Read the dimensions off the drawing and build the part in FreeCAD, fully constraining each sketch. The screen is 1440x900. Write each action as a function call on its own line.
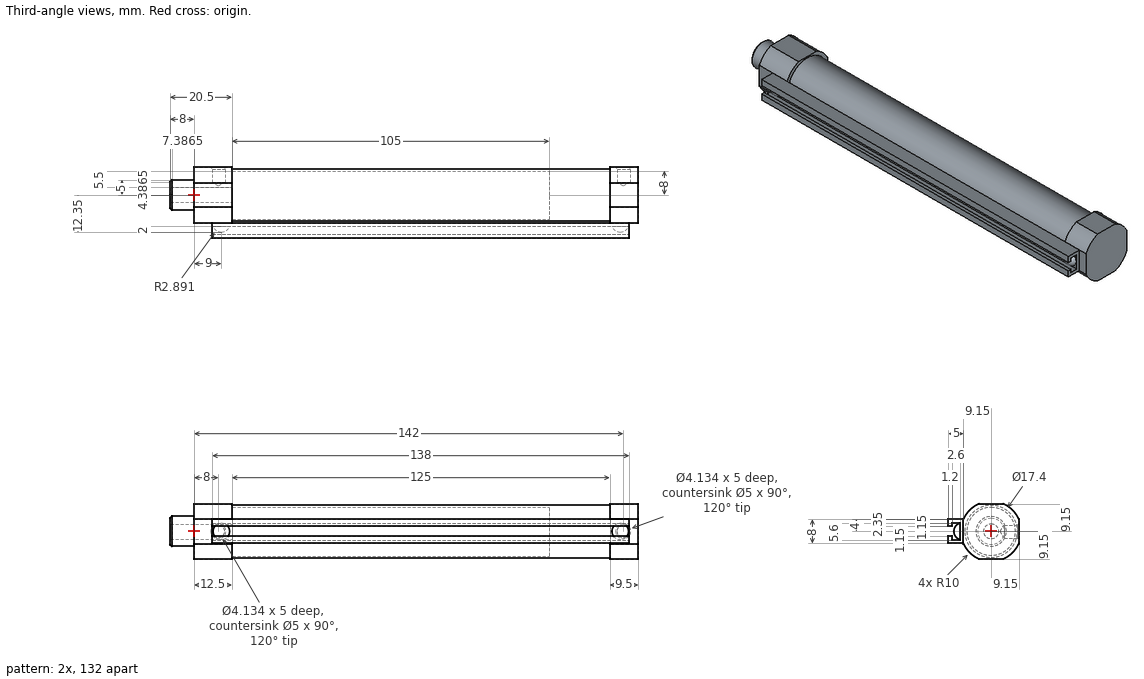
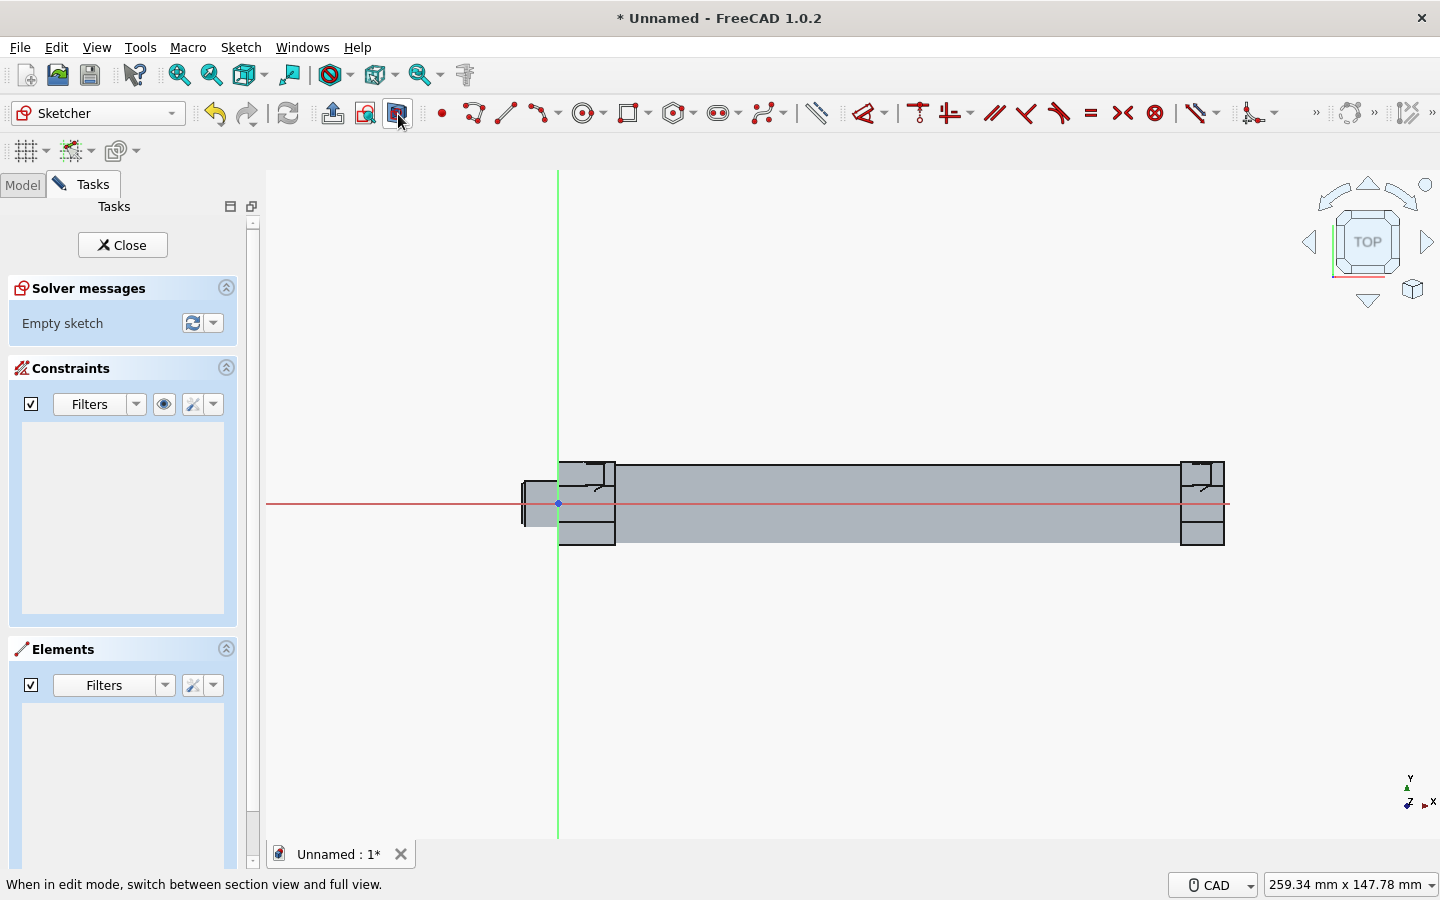
click(474, 114)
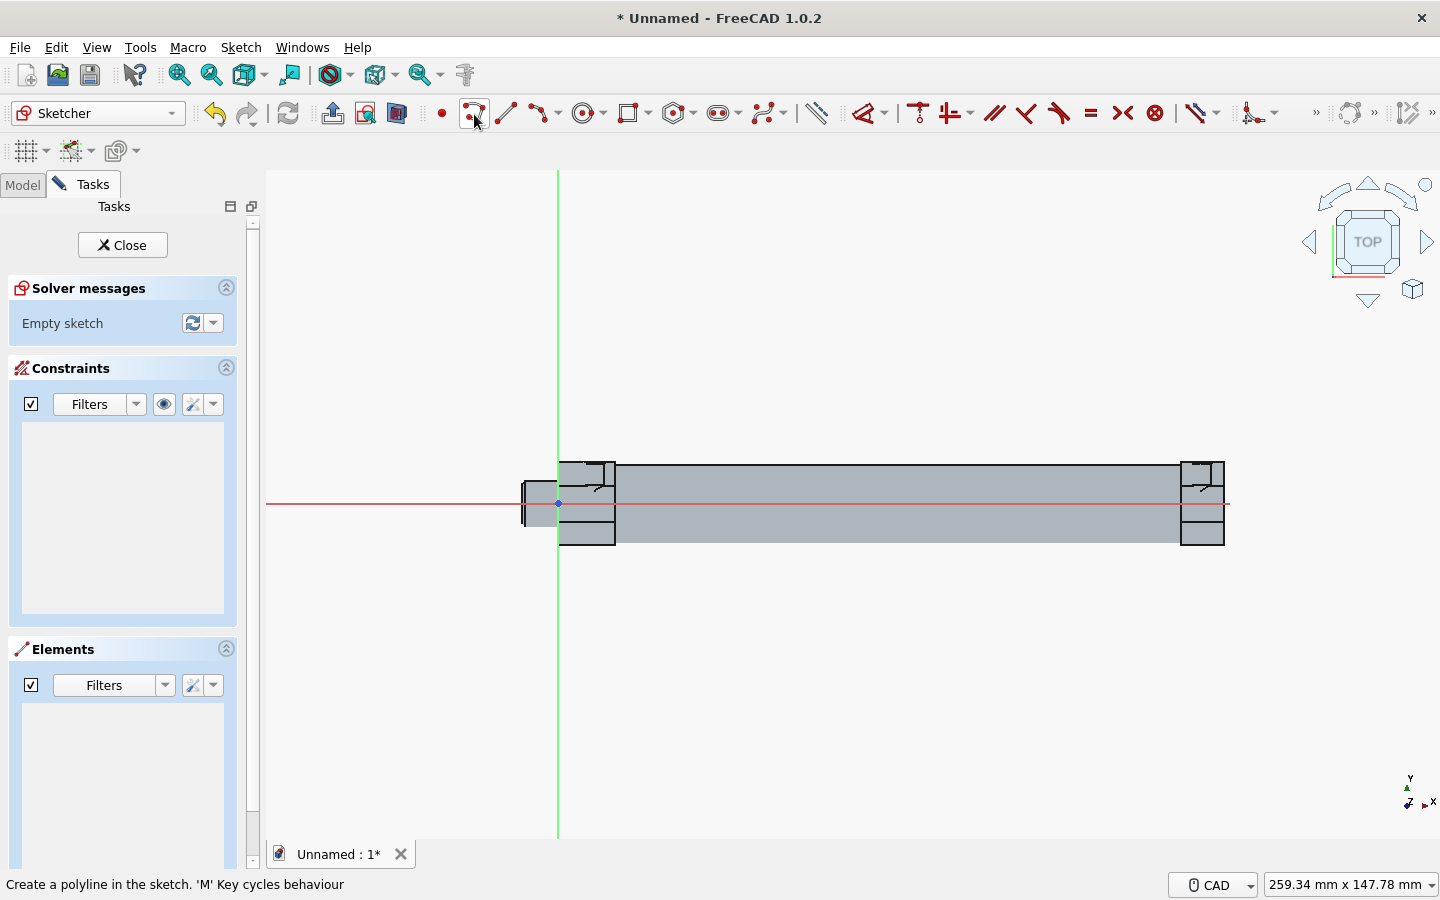
click(522, 504)
click(1090, 495)
click(1090, 468)
click(615, 468)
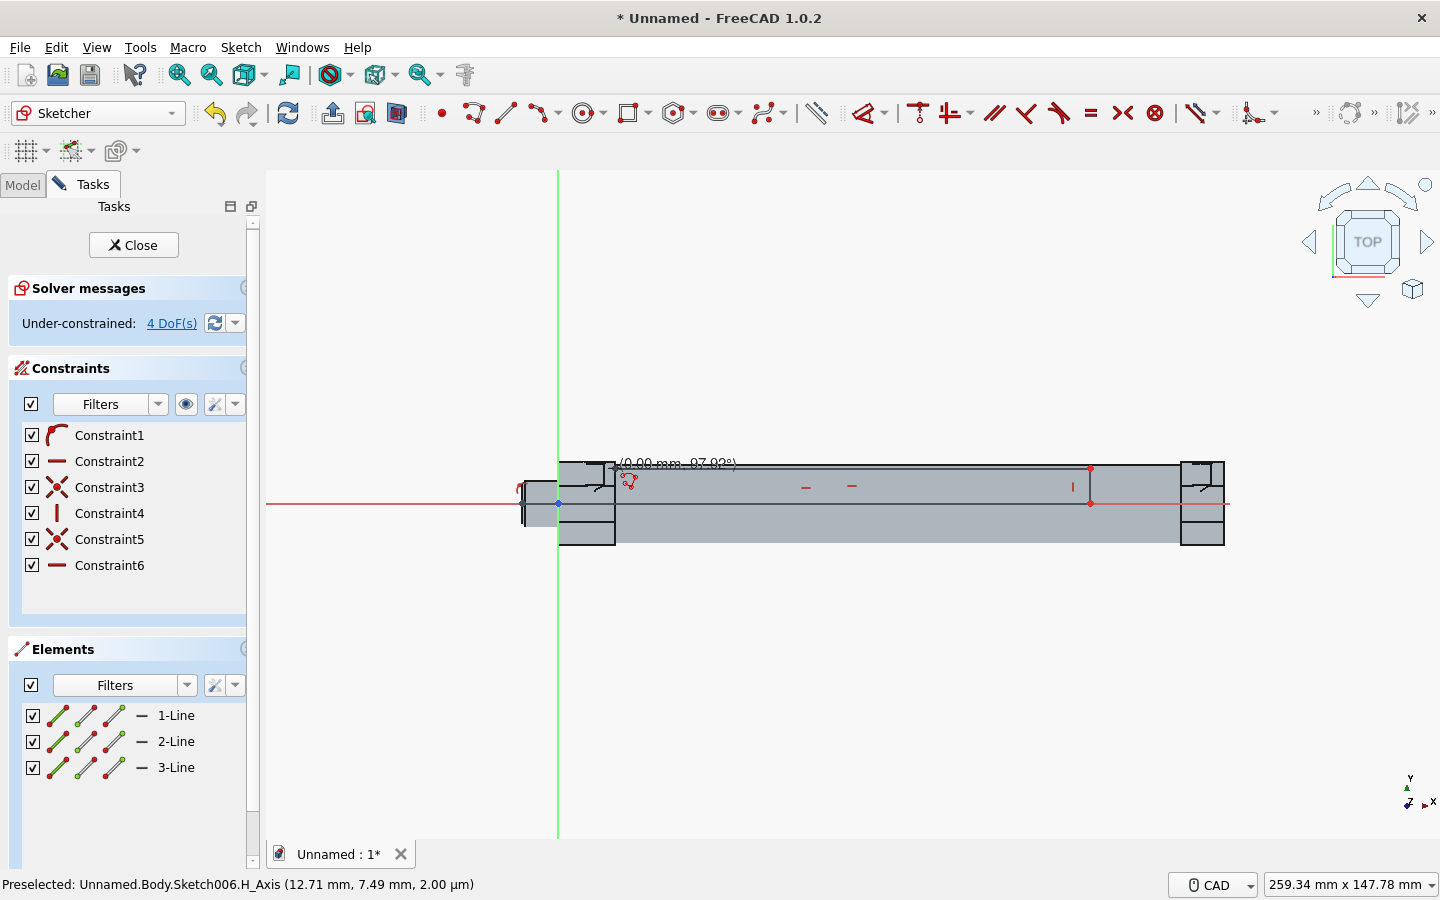
scroll(615, 493, up, 2)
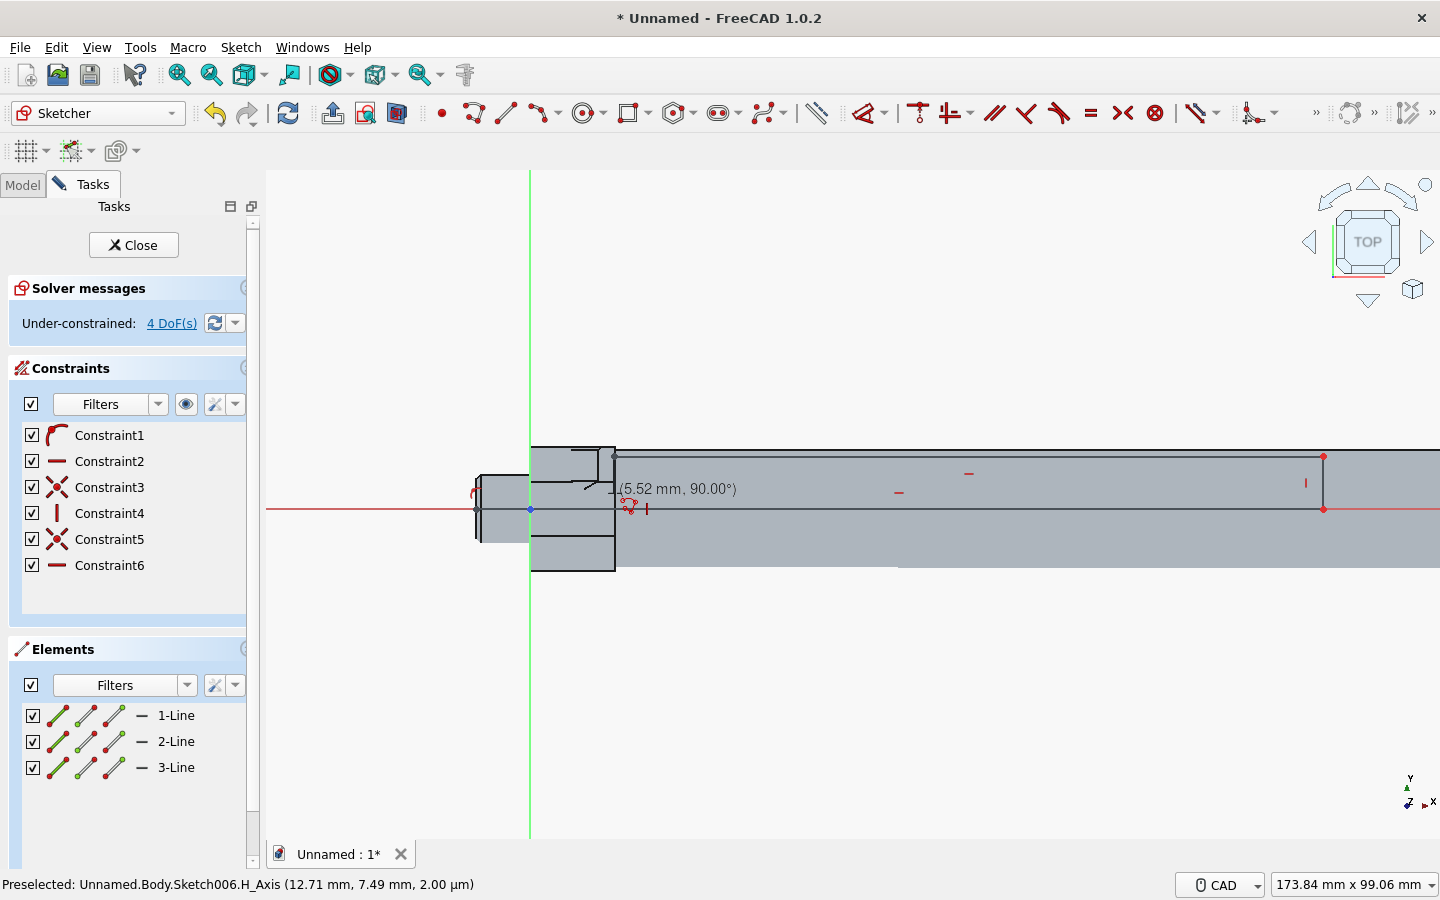
click(615, 492)
click(476, 492)
click(476, 509)
key(Escape)
key(Escape)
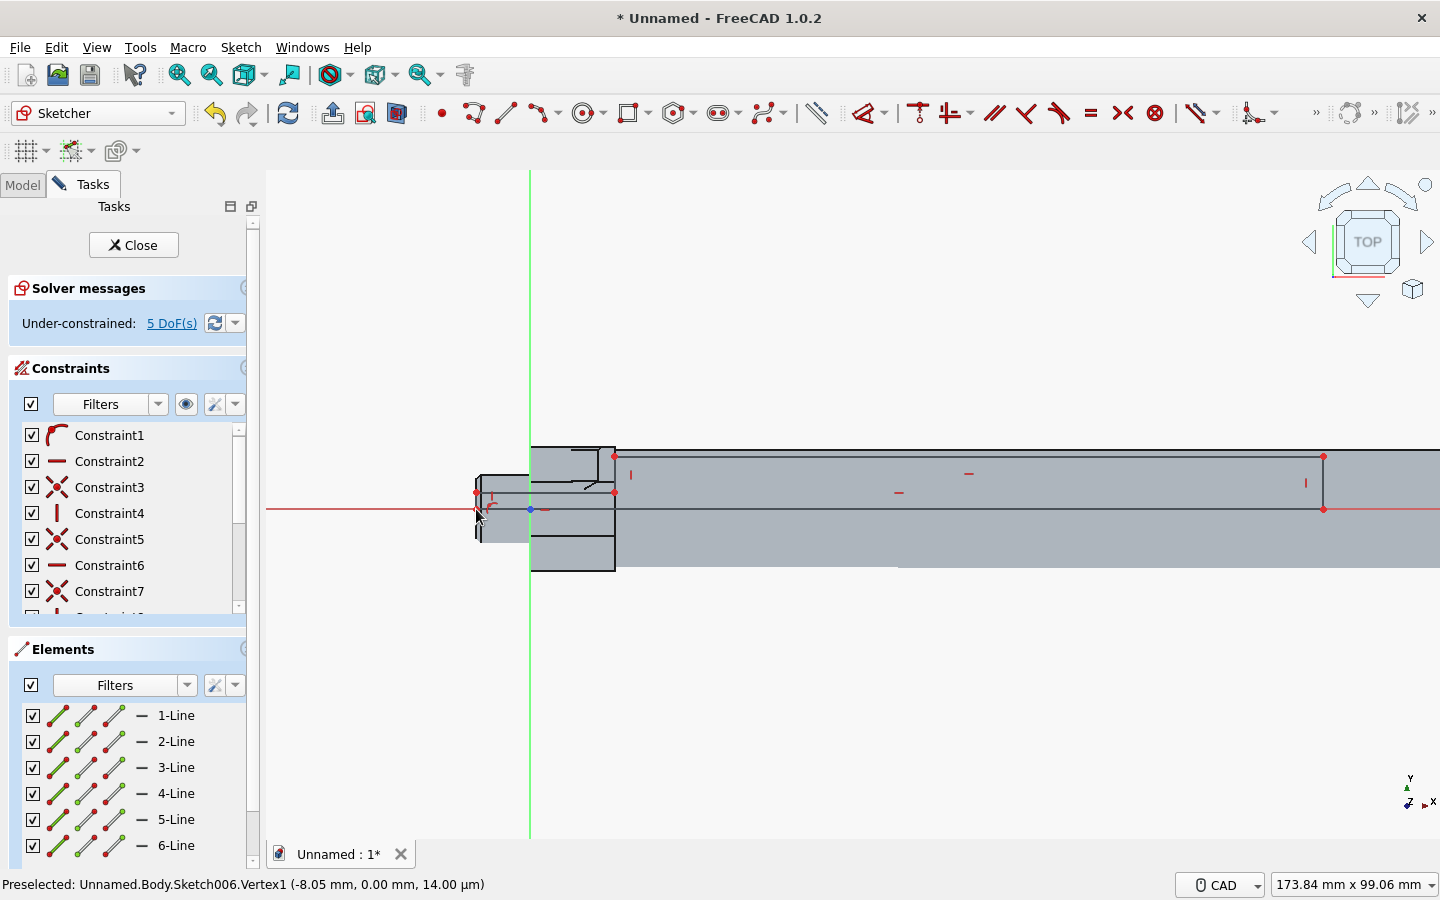
click(864, 114)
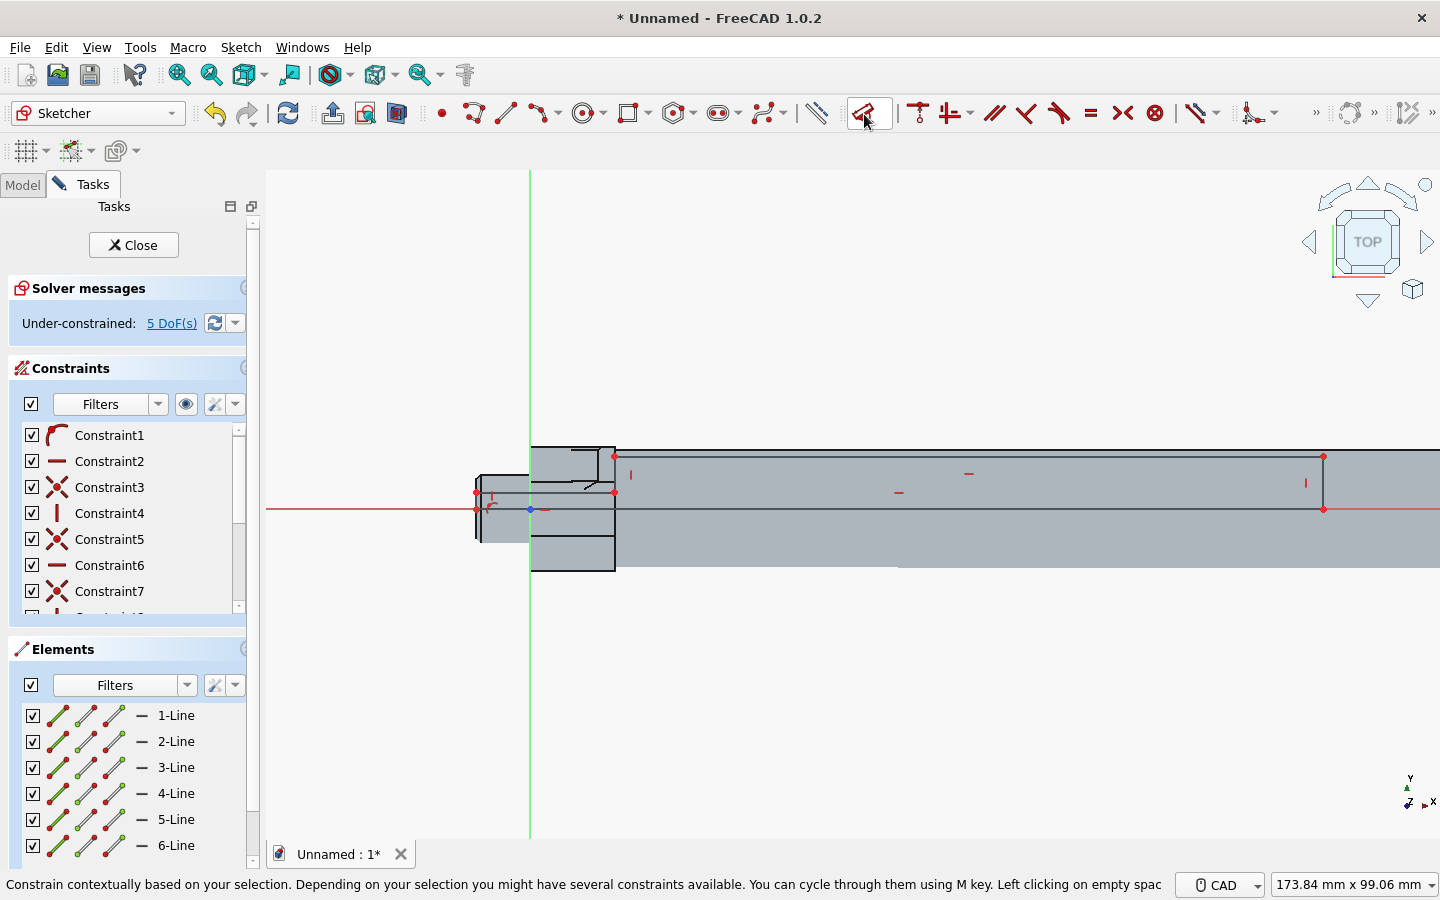
scroll(294, 606, down, 1)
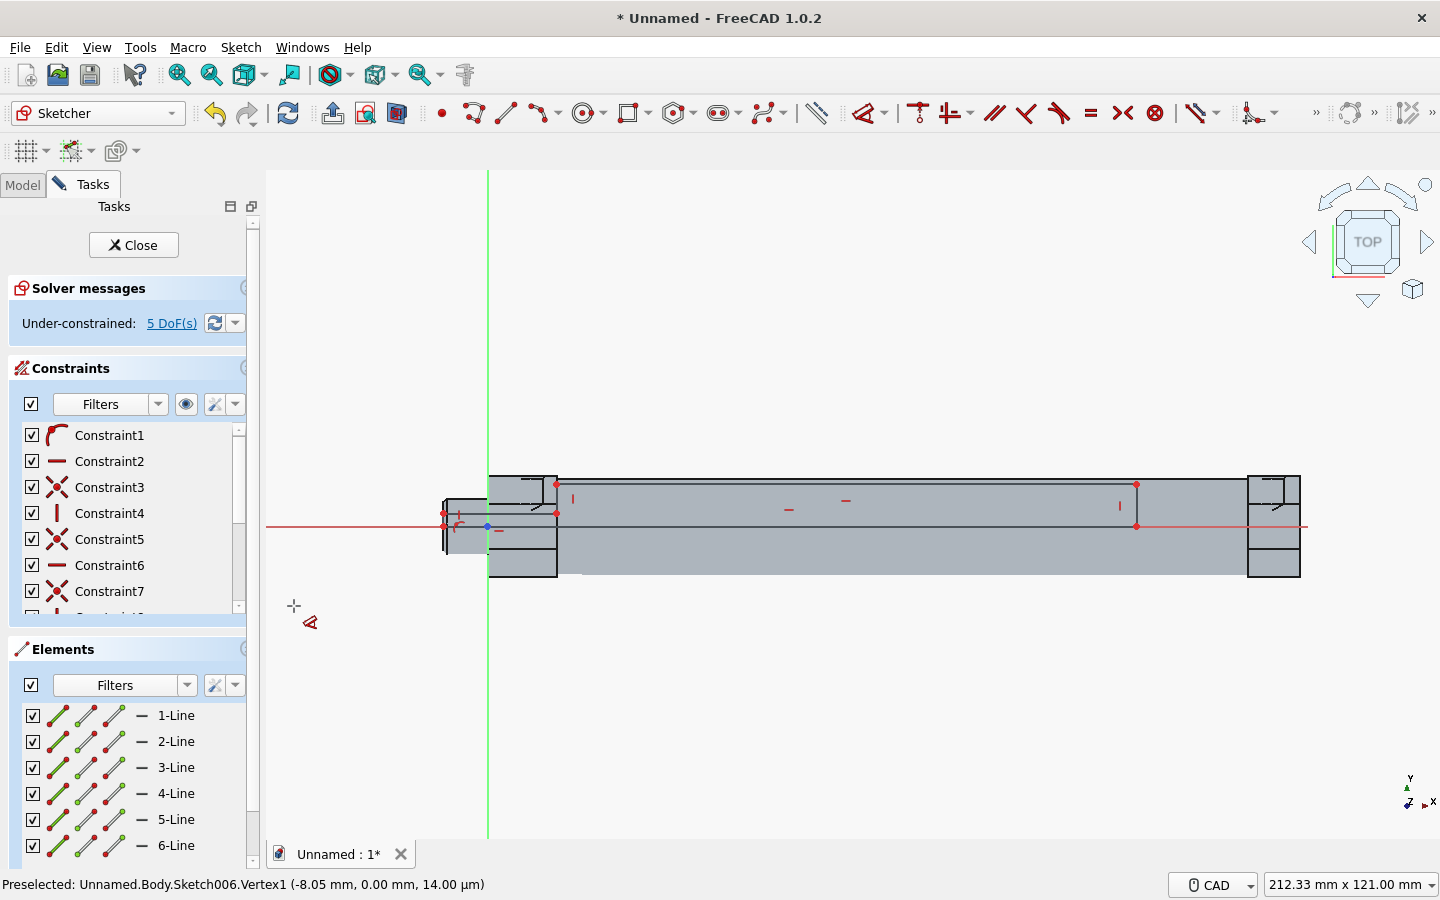
click(1137, 514)
click(1171, 505)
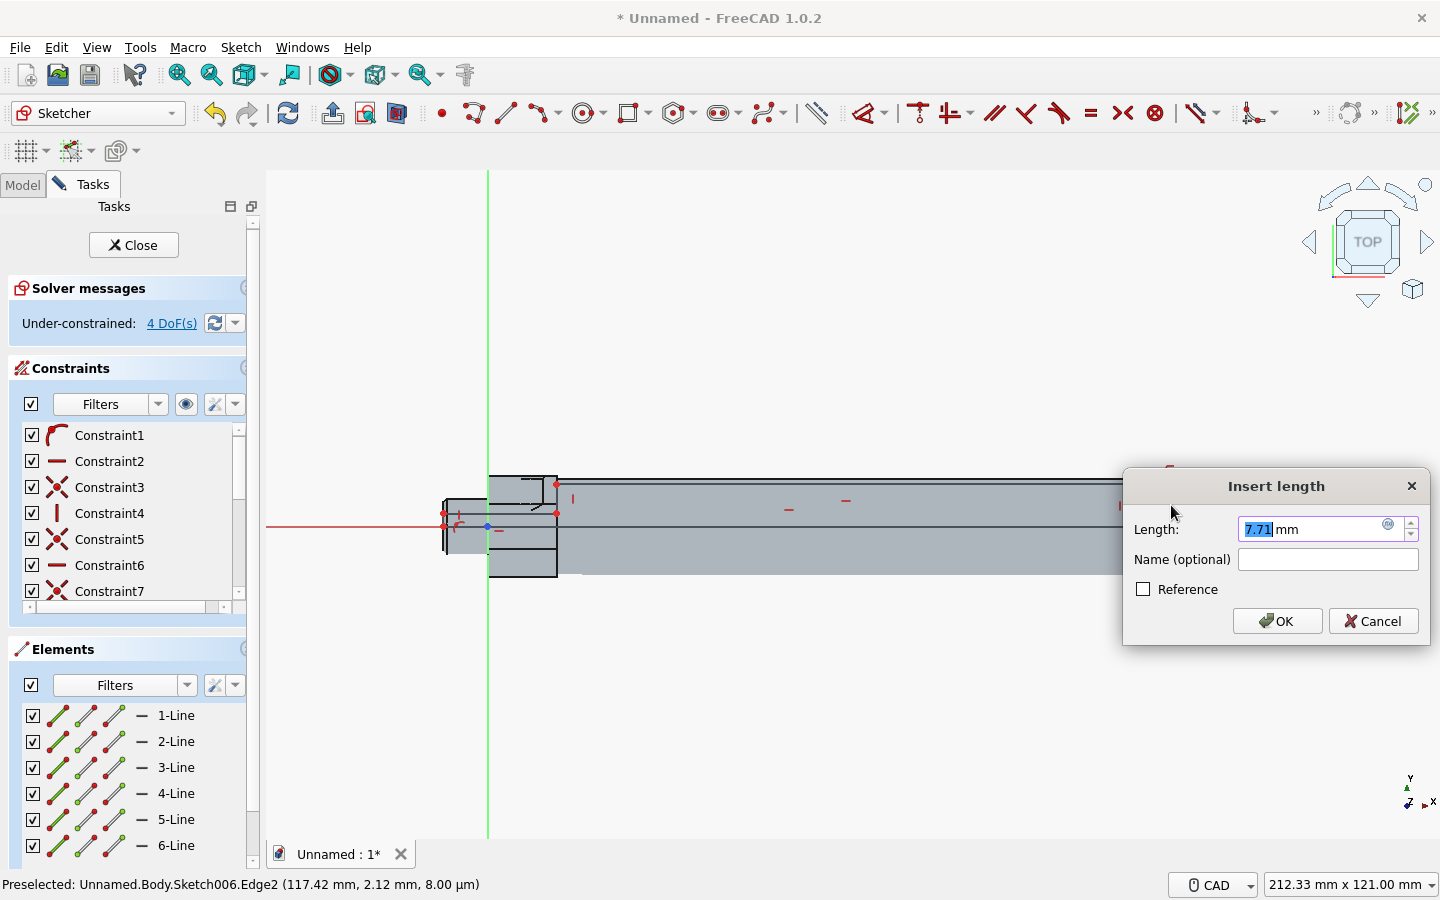
text(8)
key(Return)